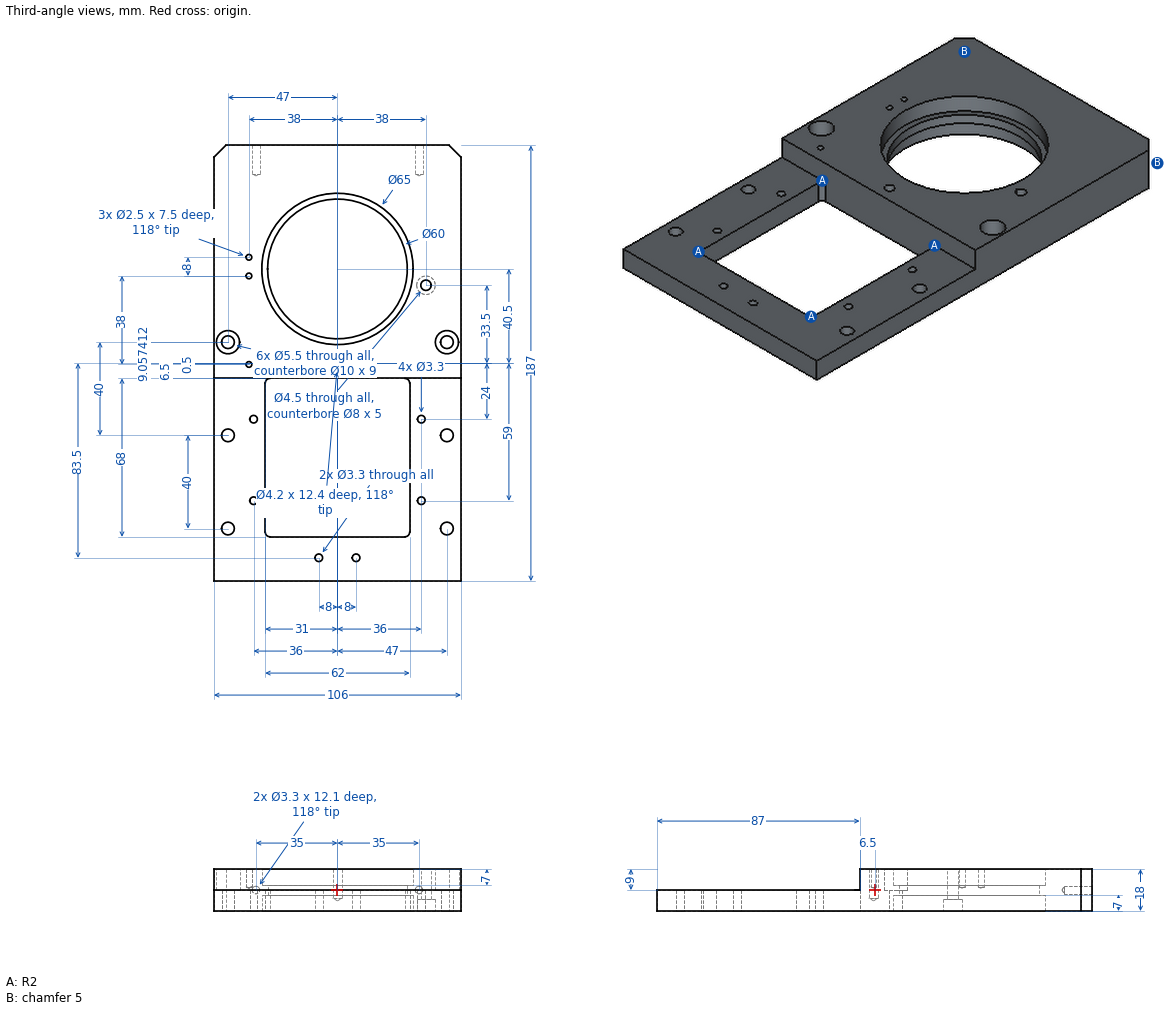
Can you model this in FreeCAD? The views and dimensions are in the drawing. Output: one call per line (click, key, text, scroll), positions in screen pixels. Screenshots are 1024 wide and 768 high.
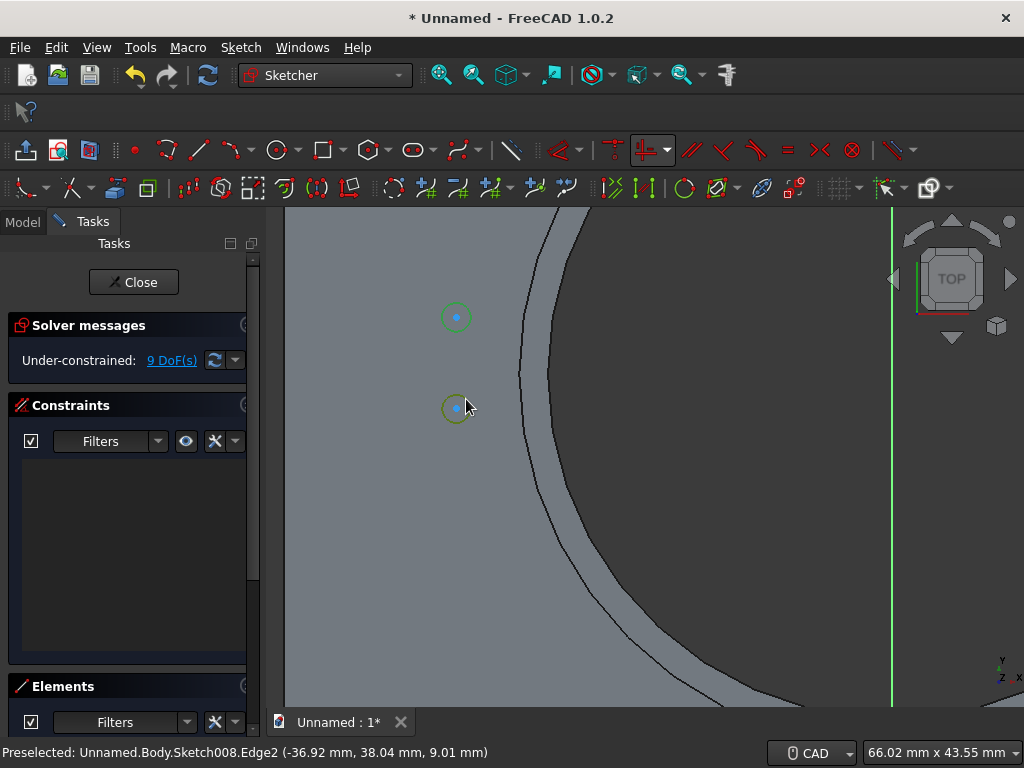
scroll(466, 307, down, 3)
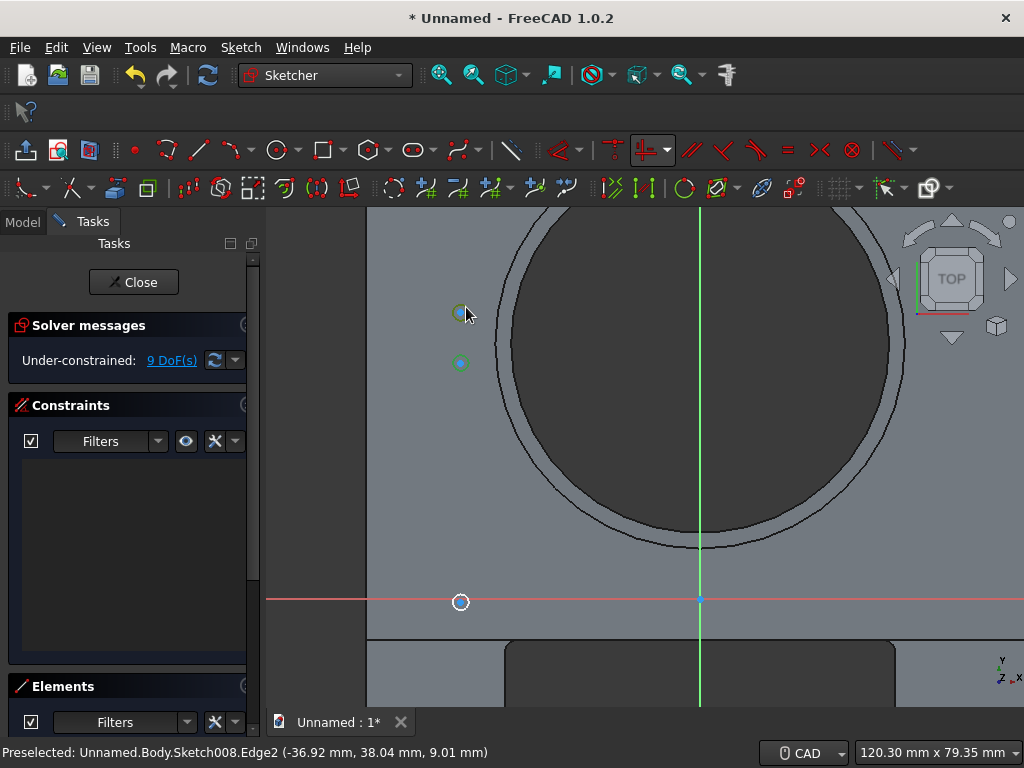
scroll(455, 608, up, 3)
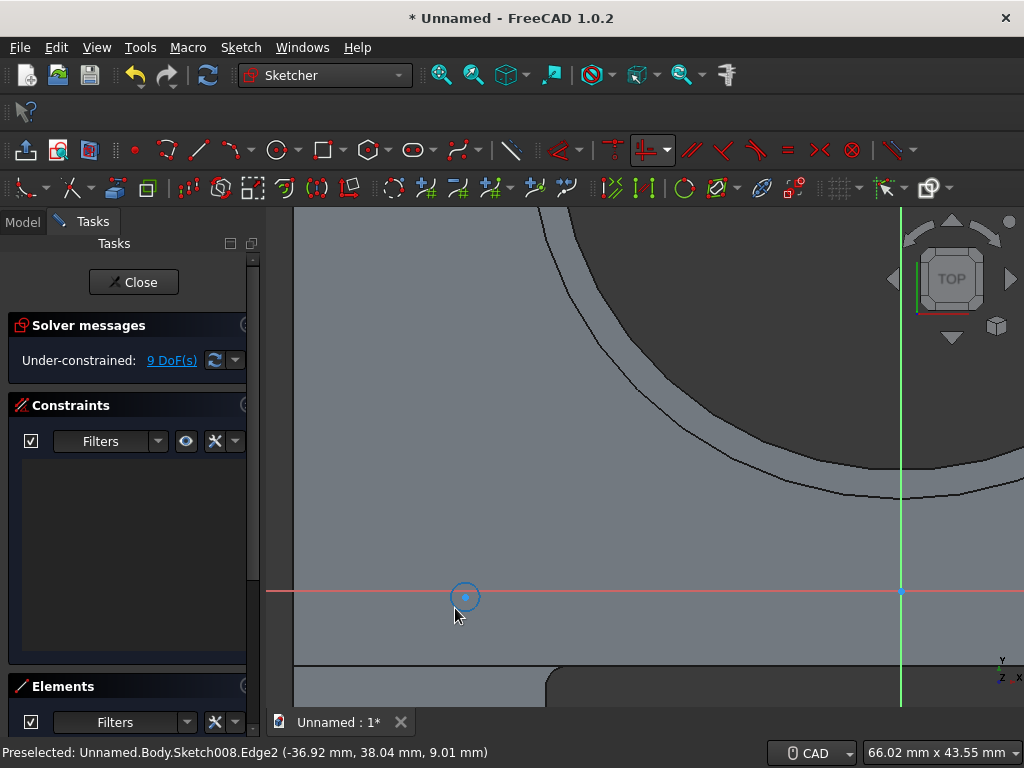
click(455, 607)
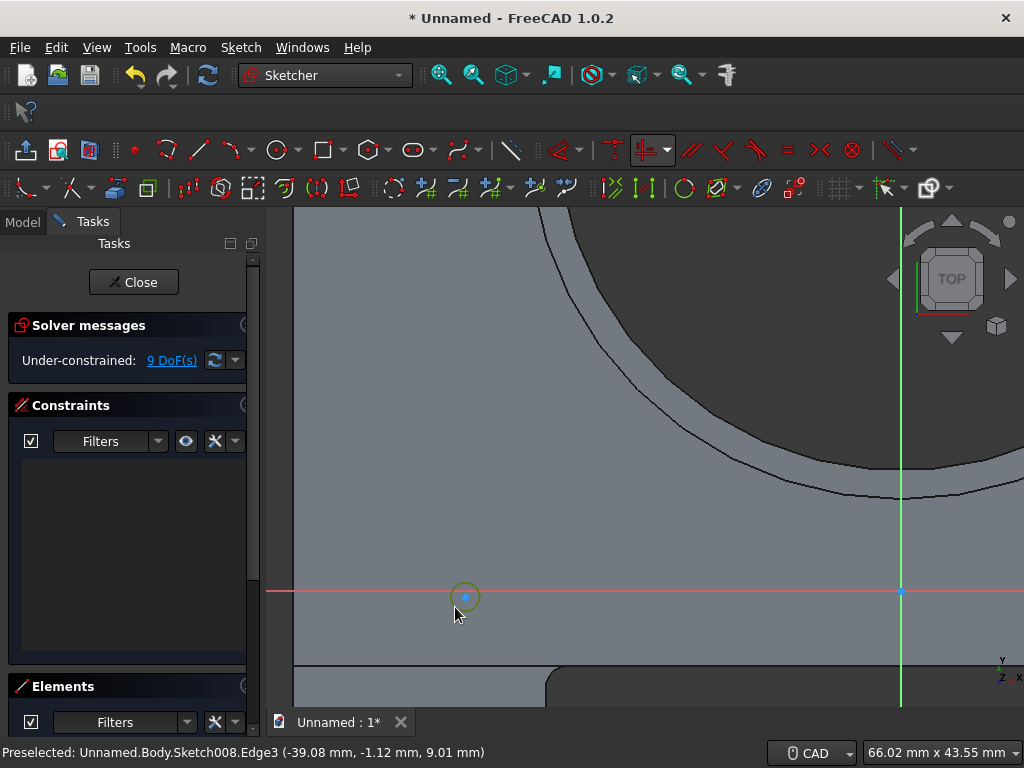
click(788, 150)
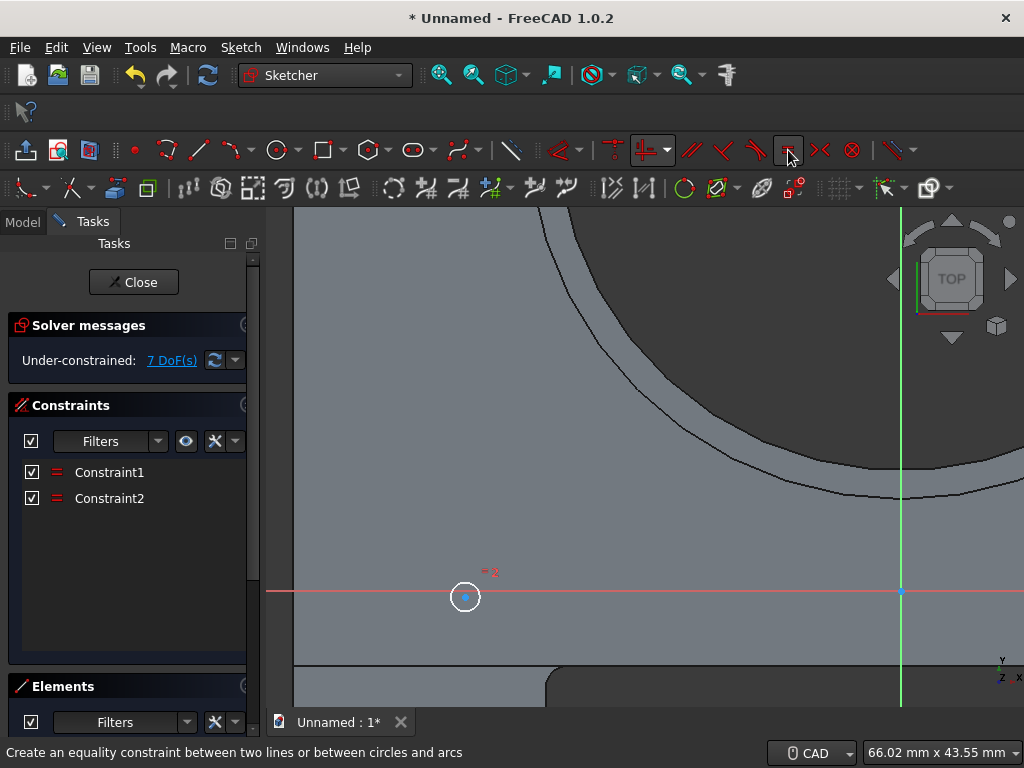
scroll(455, 608, down, 3)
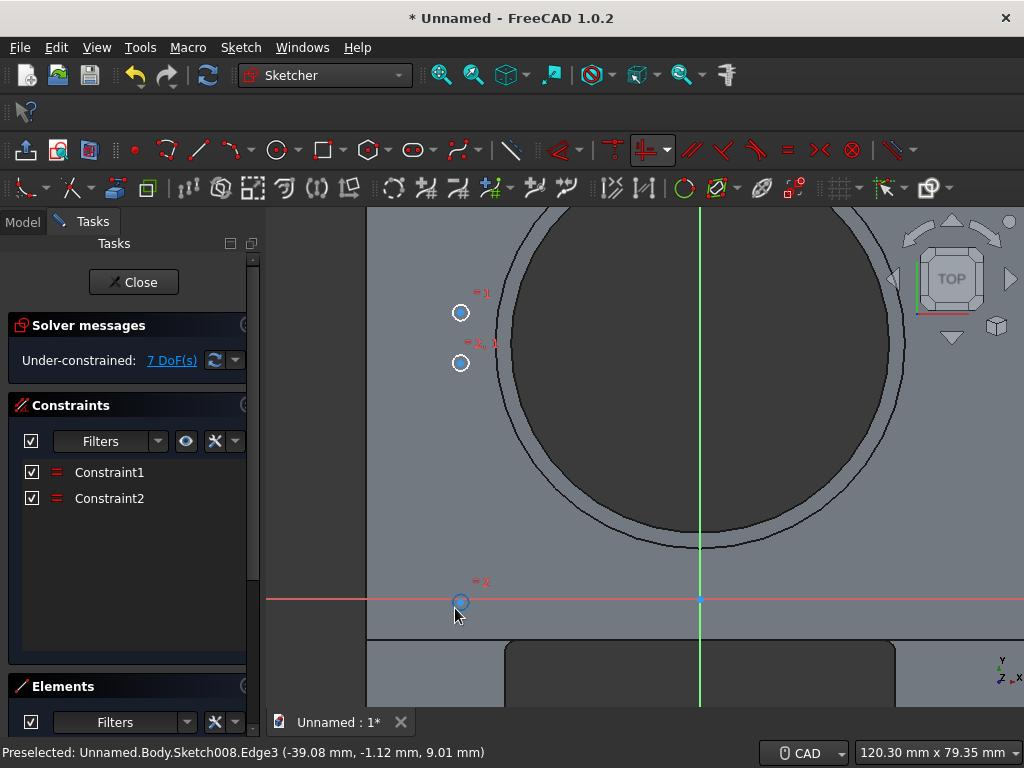
click(461, 313)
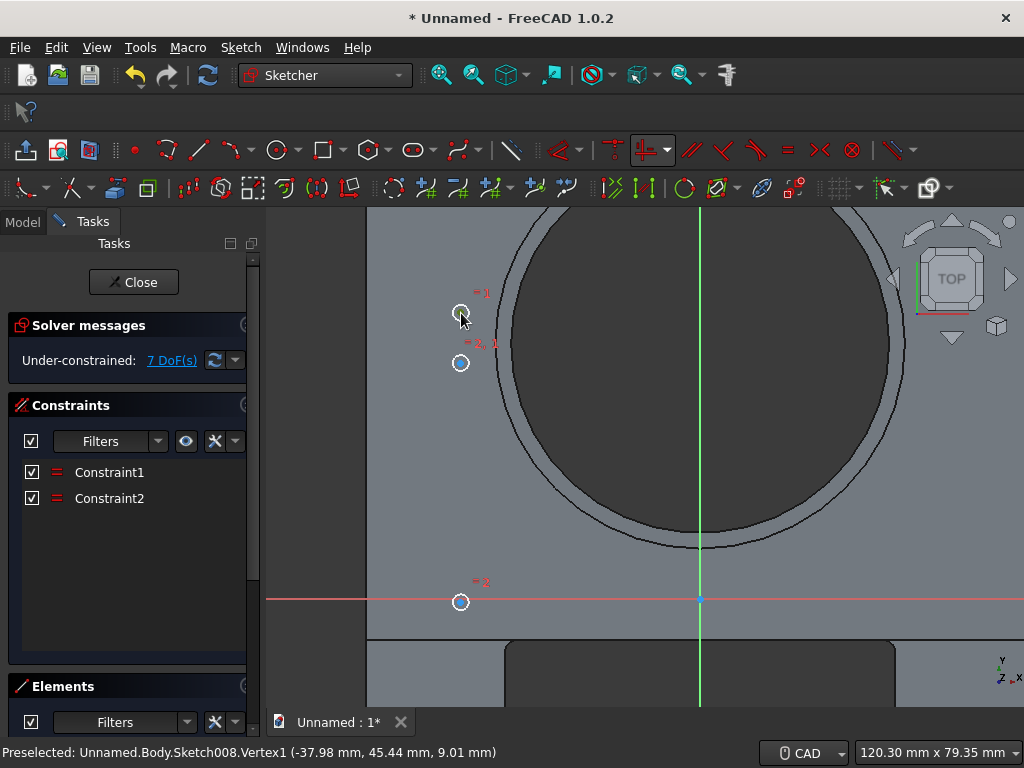
click(461, 363)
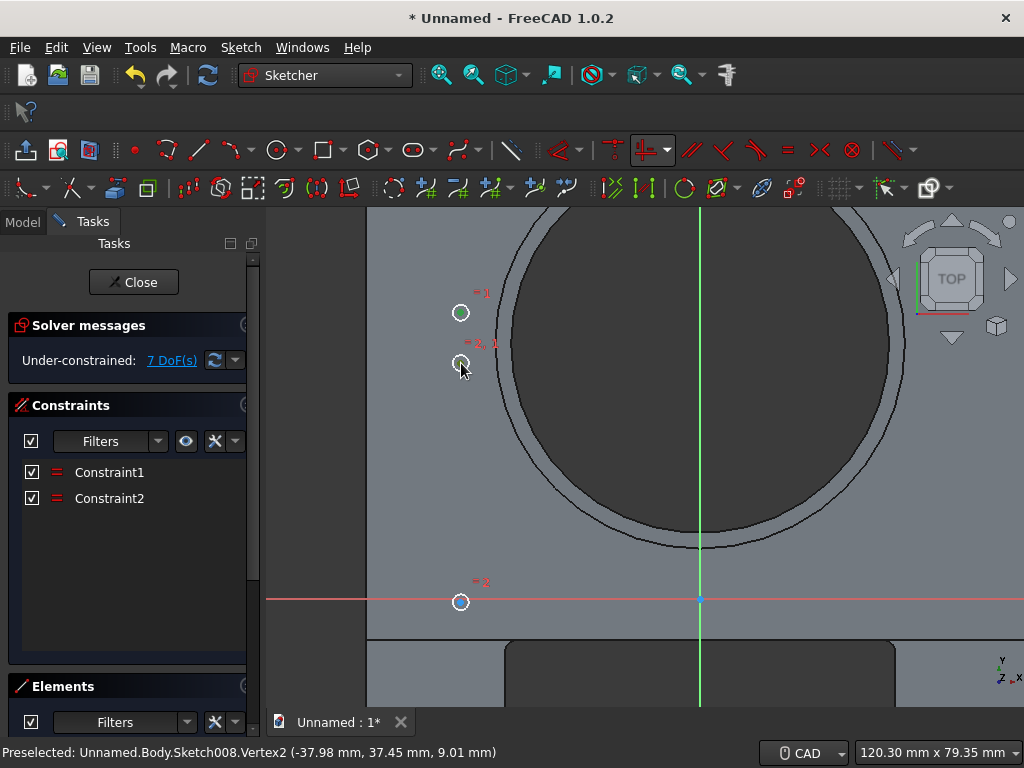
click(670, 150)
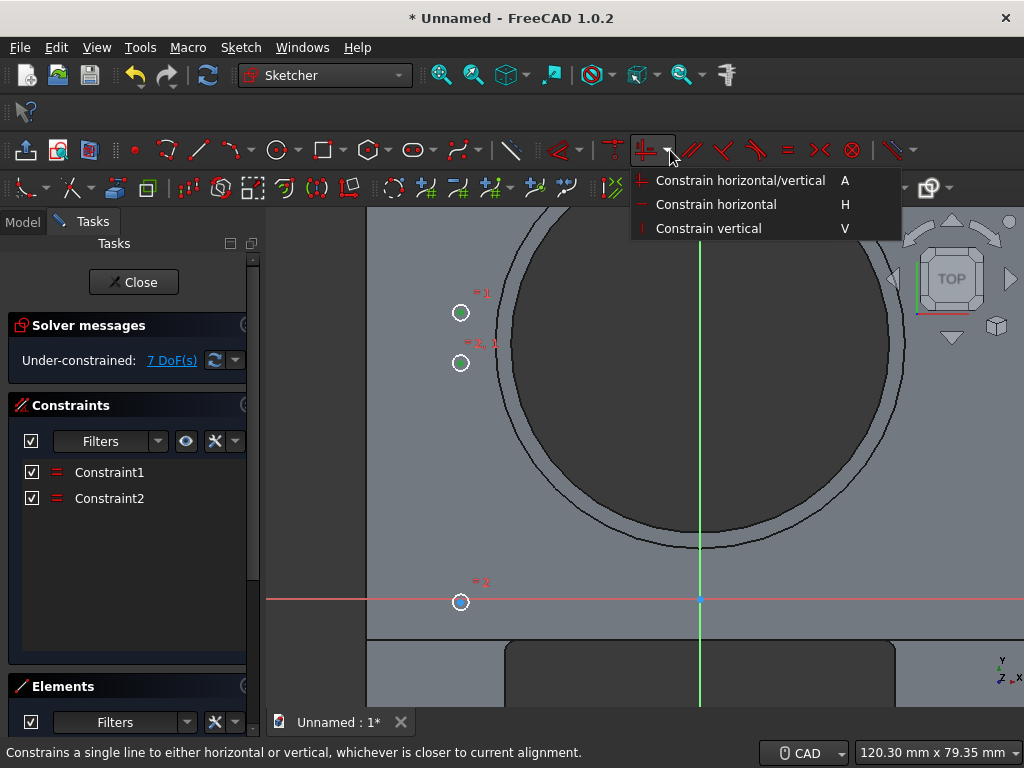
click(766, 228)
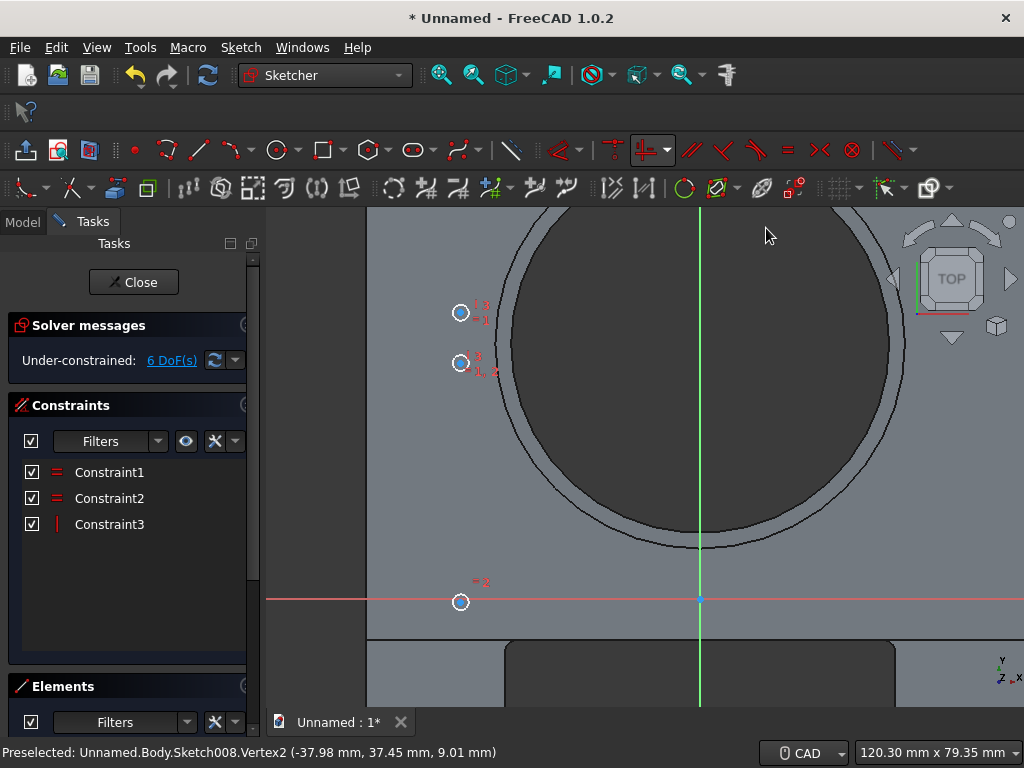
click(461, 363)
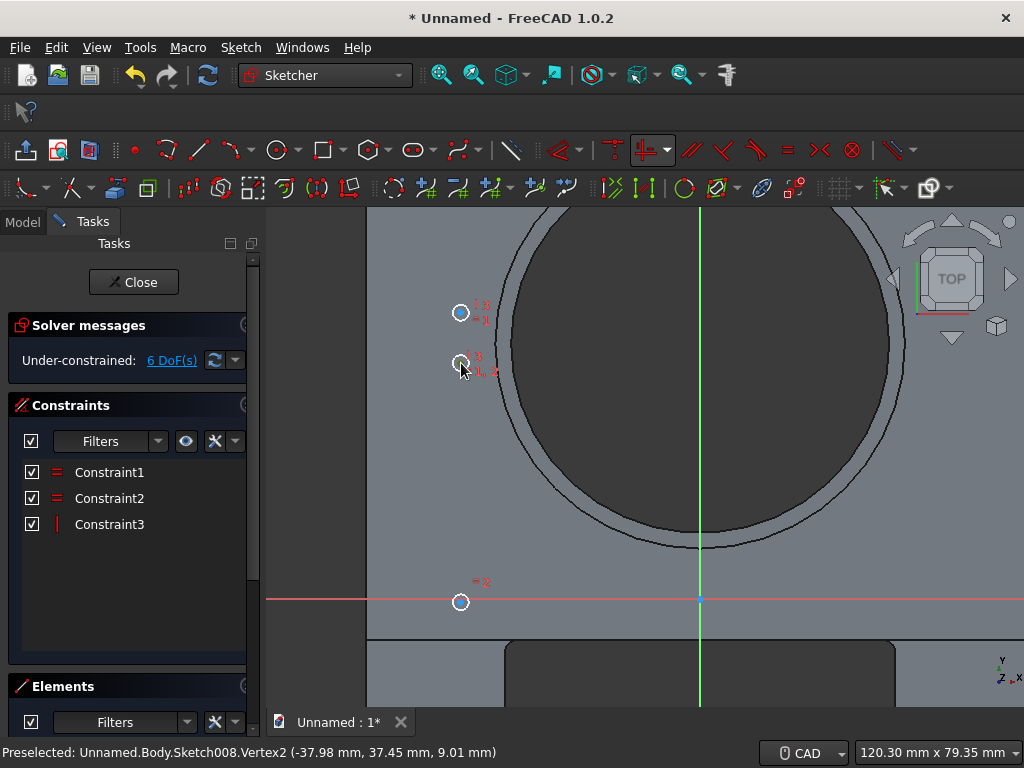
click(461, 602)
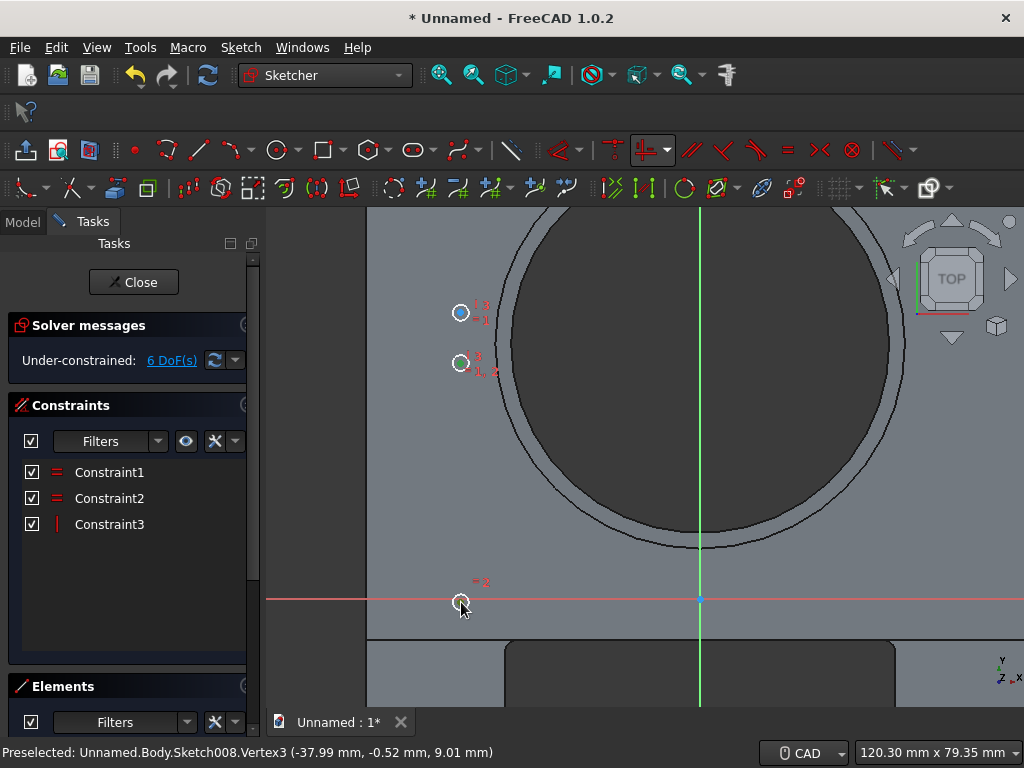
click(670, 150)